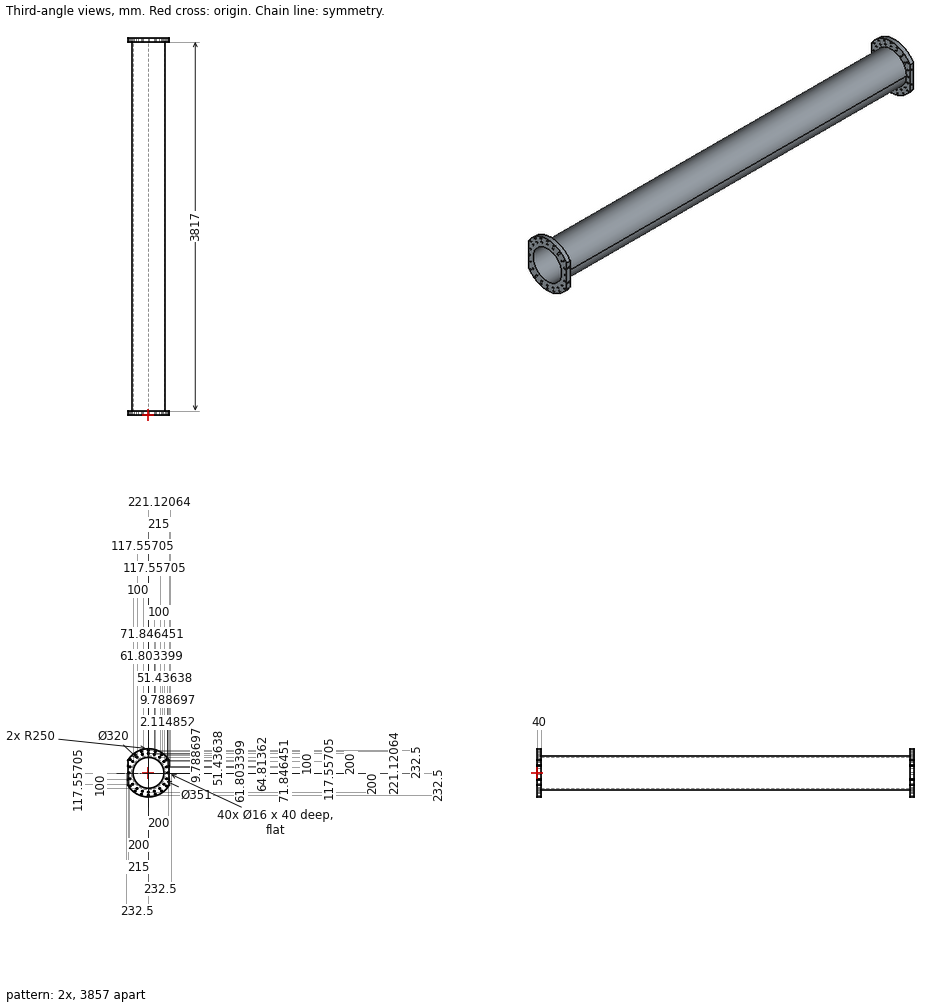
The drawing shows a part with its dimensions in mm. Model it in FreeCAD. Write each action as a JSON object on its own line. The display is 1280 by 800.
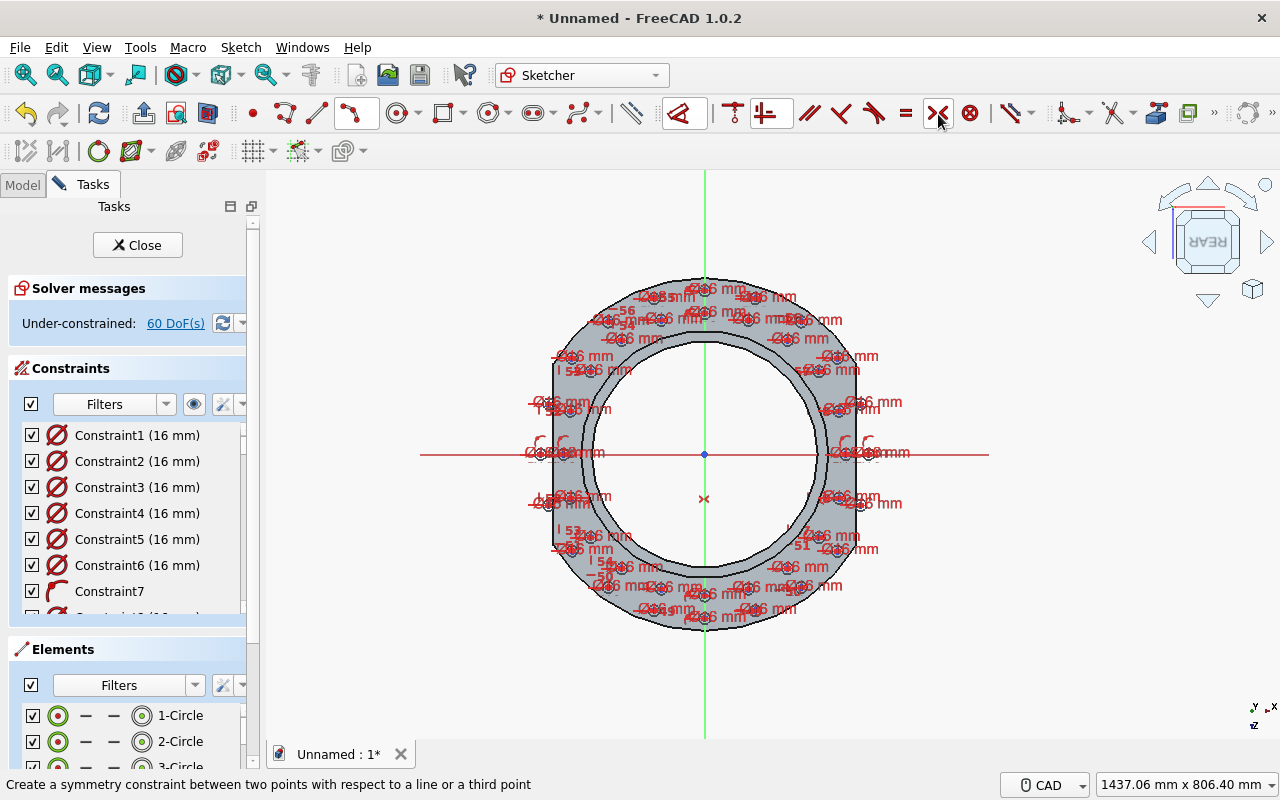
{"action": "left_click", "coordinate": [661, 589]}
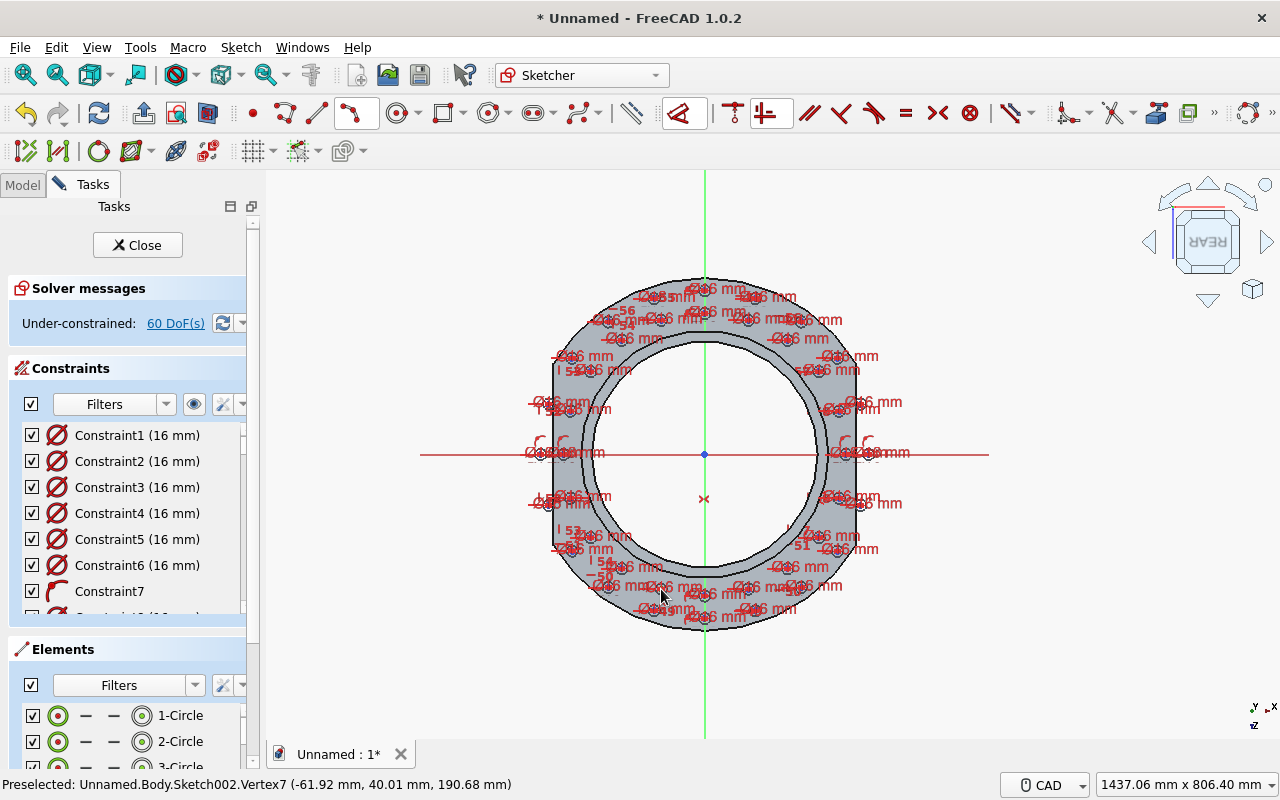
{"action": "left_click", "coordinate": [661, 320]}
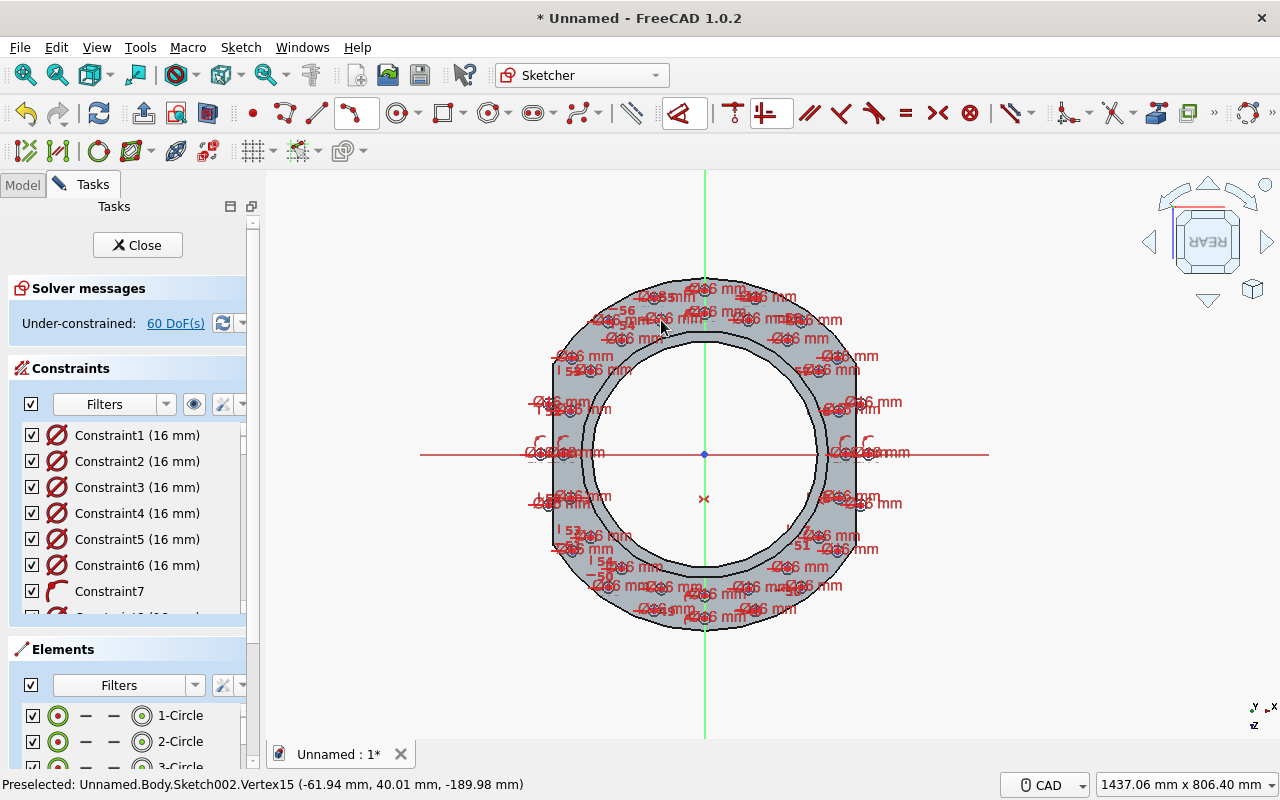
{"action": "left_click", "coordinate": [470, 454]}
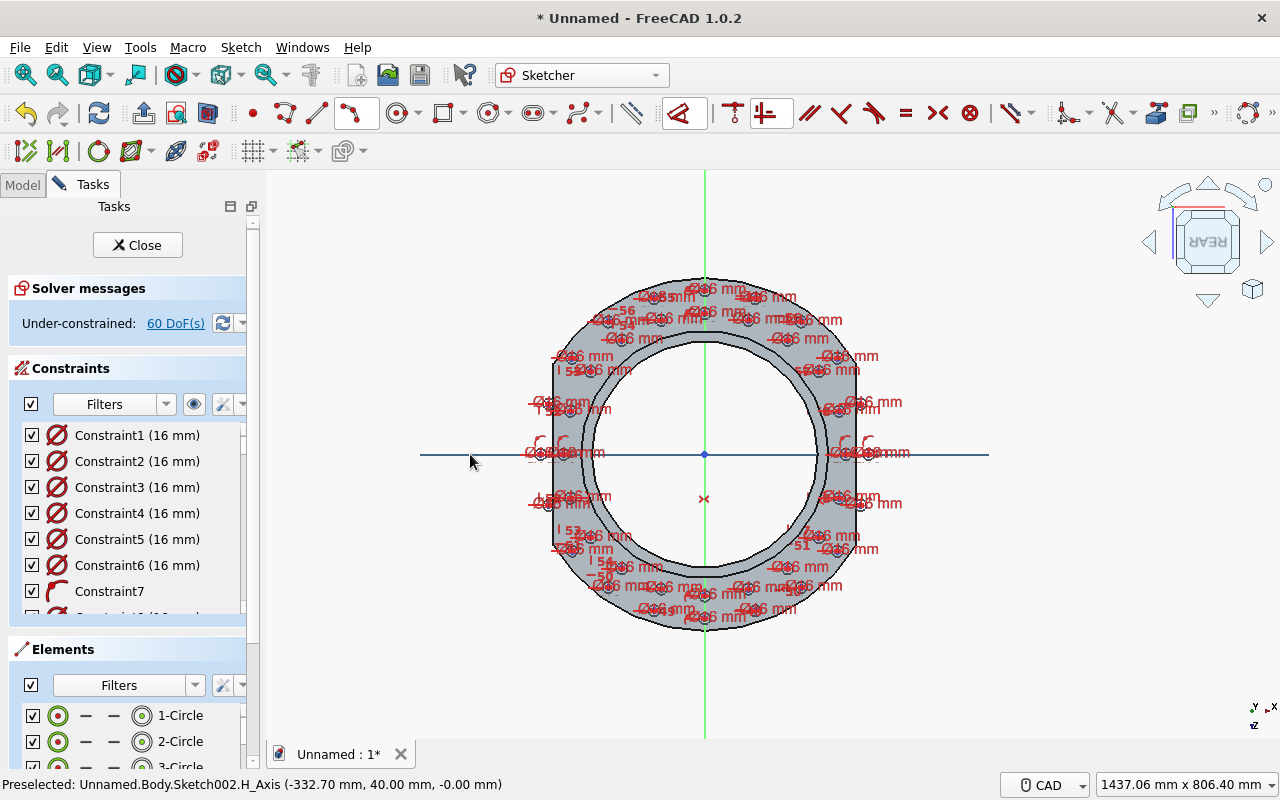
{"action": "left_click", "coordinate": [938, 114]}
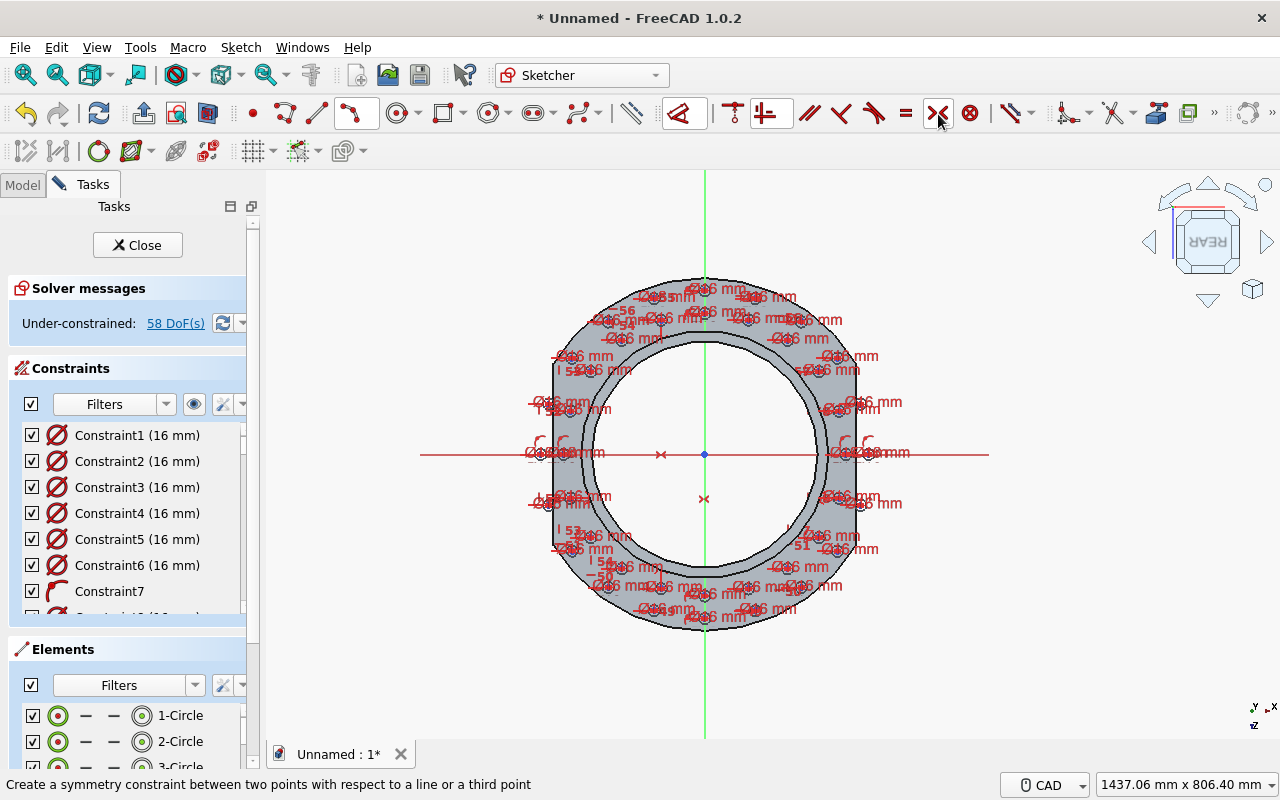
{"action": "left_click", "coordinate": [788, 569]}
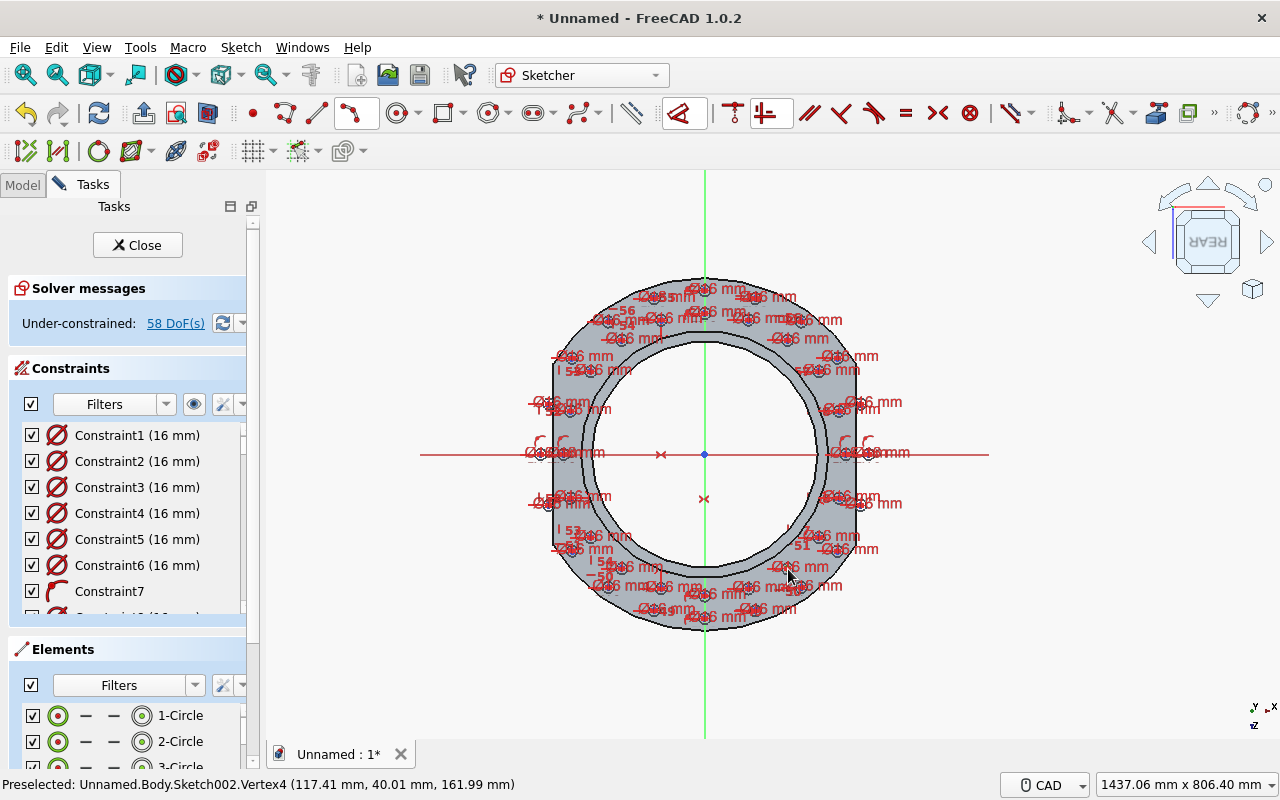
{"action": "left_click", "coordinate": [788, 340]}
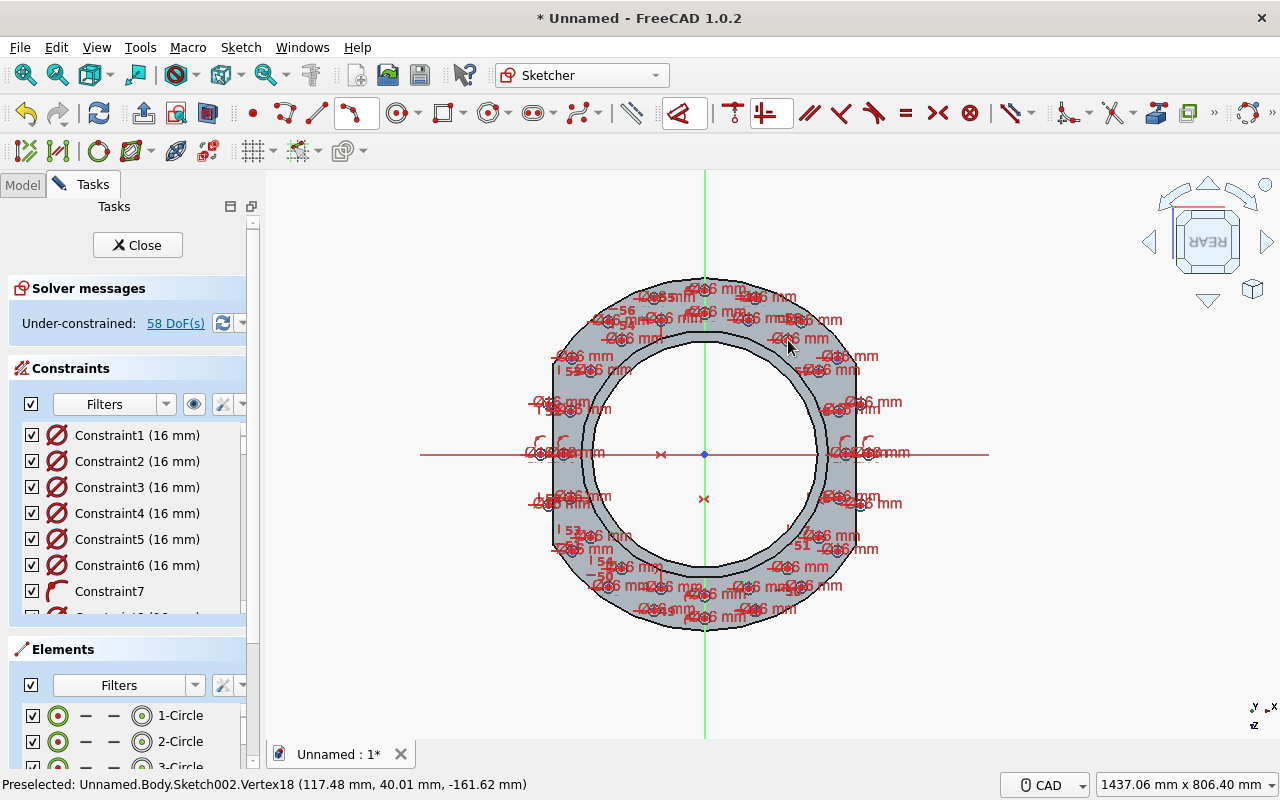
{"action": "left_click", "coordinate": [470, 454]}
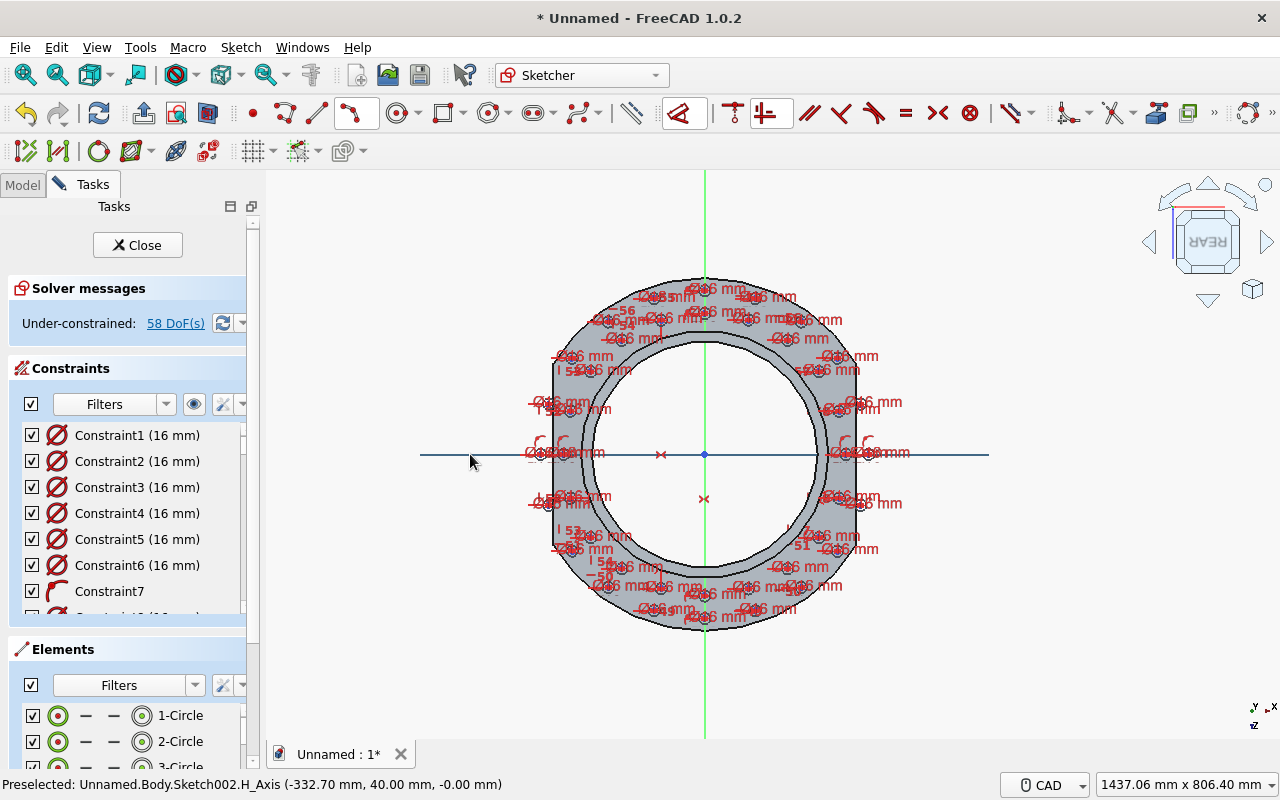
{"action": "left_click", "coordinate": [938, 114]}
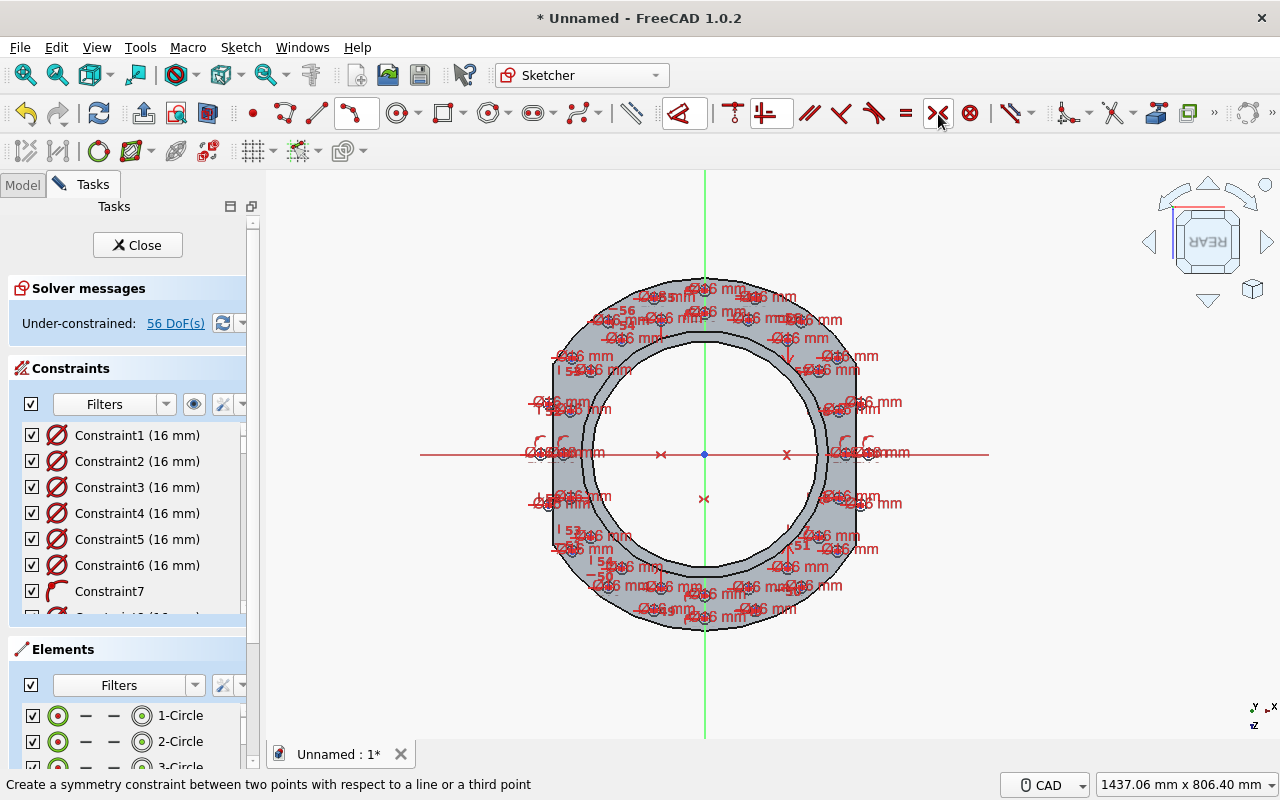
{"action": "left_click", "coordinate": [591, 372]}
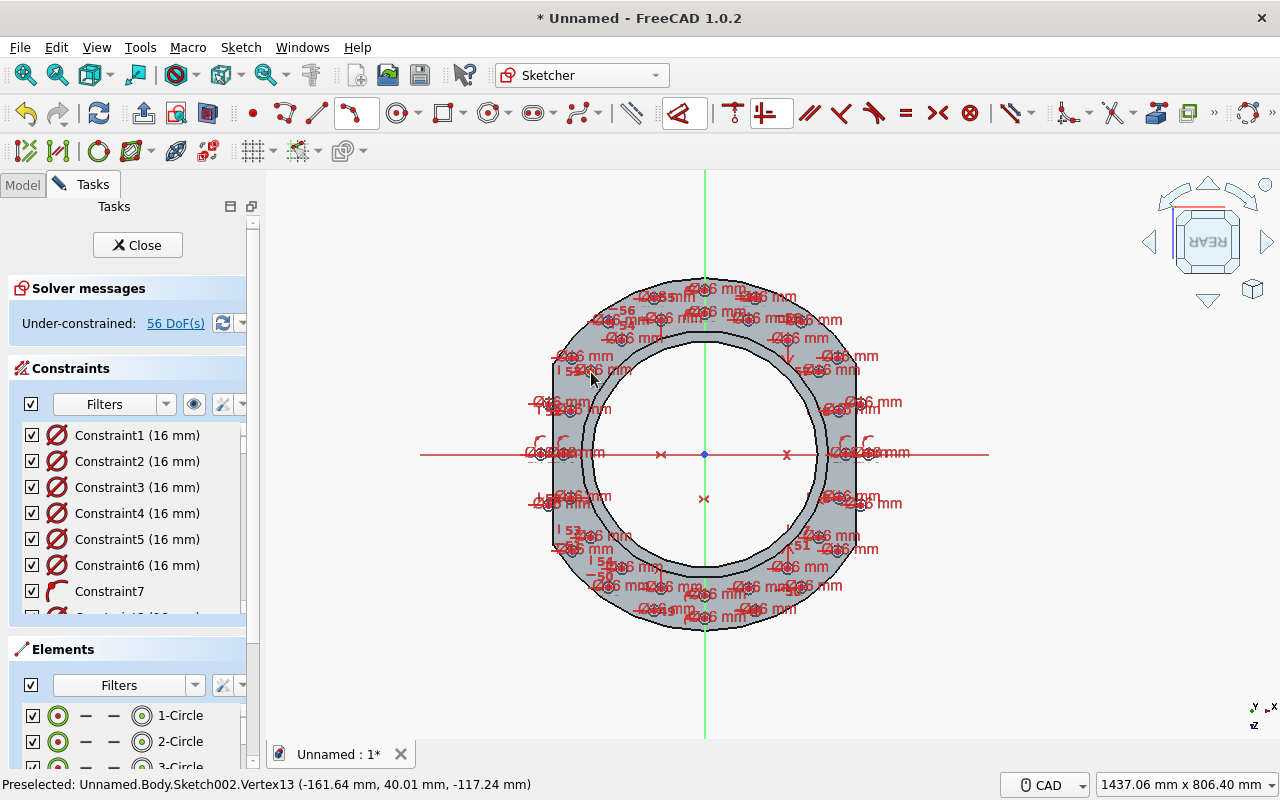
{"action": "left_click", "coordinate": [819, 372]}